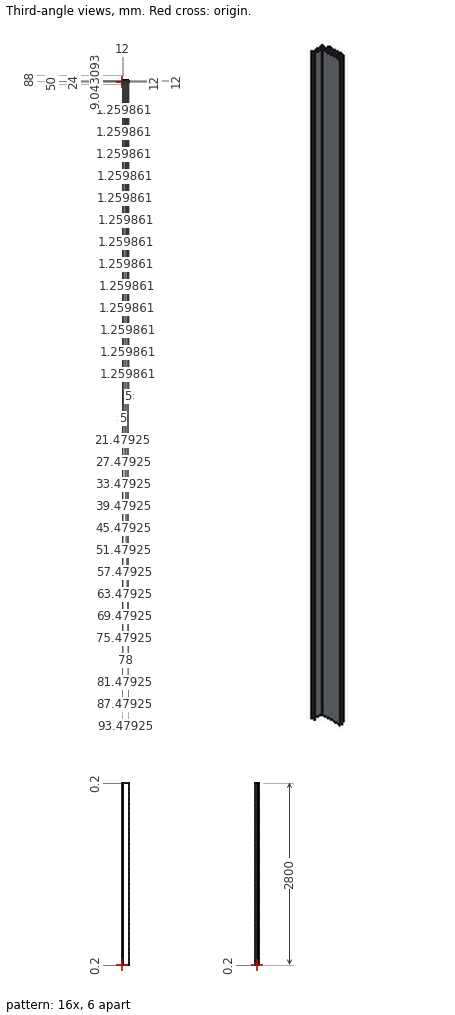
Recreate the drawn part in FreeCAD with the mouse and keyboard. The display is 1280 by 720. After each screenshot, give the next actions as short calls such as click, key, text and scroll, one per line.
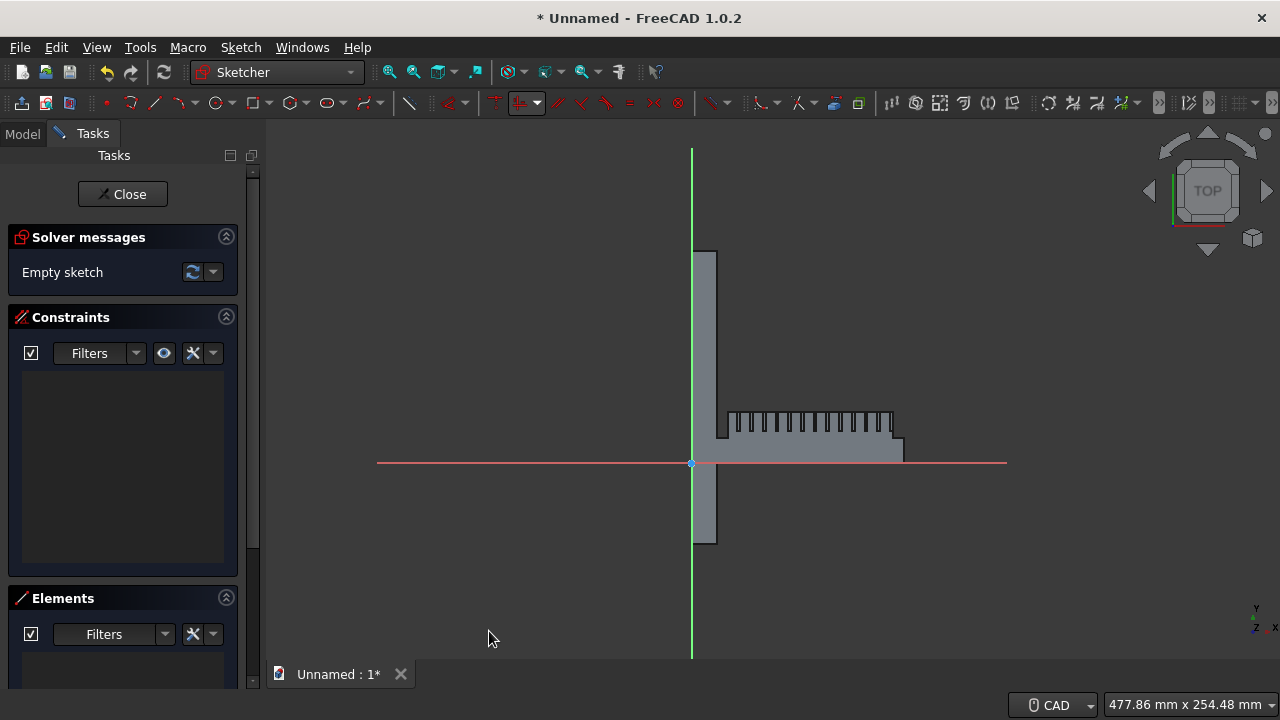
scroll(705, 292, up, 2)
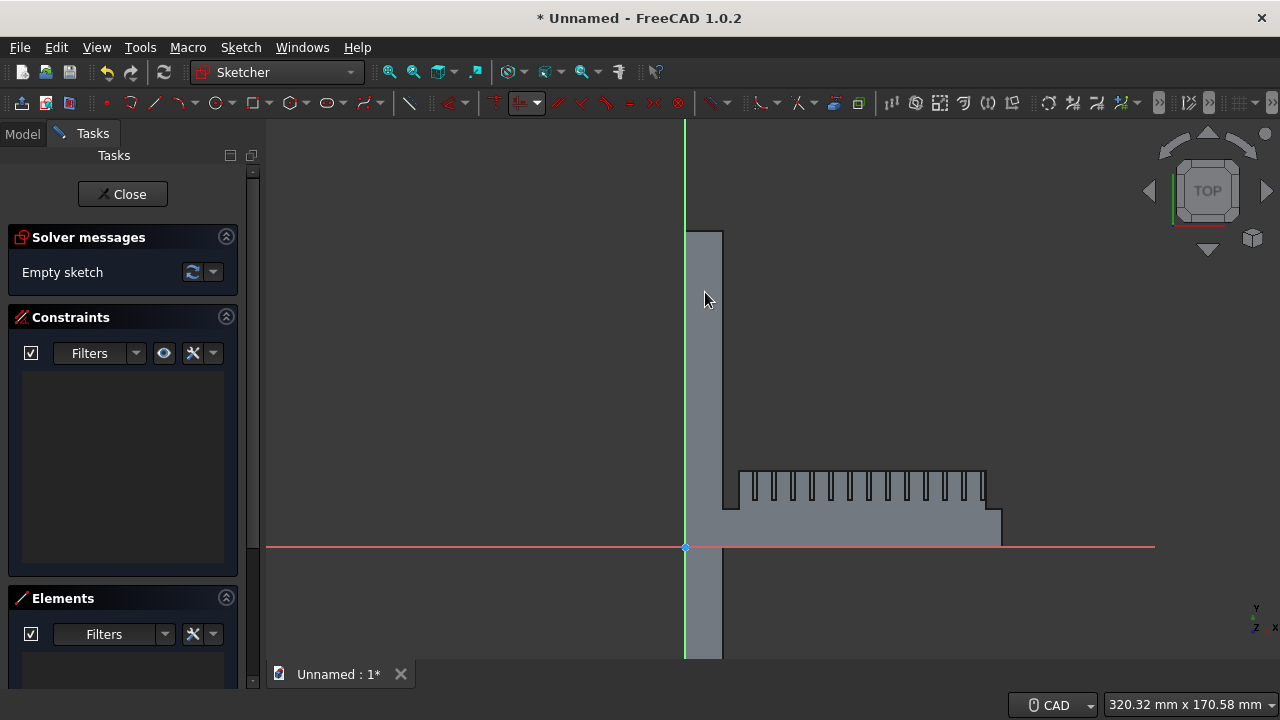
click(254, 104)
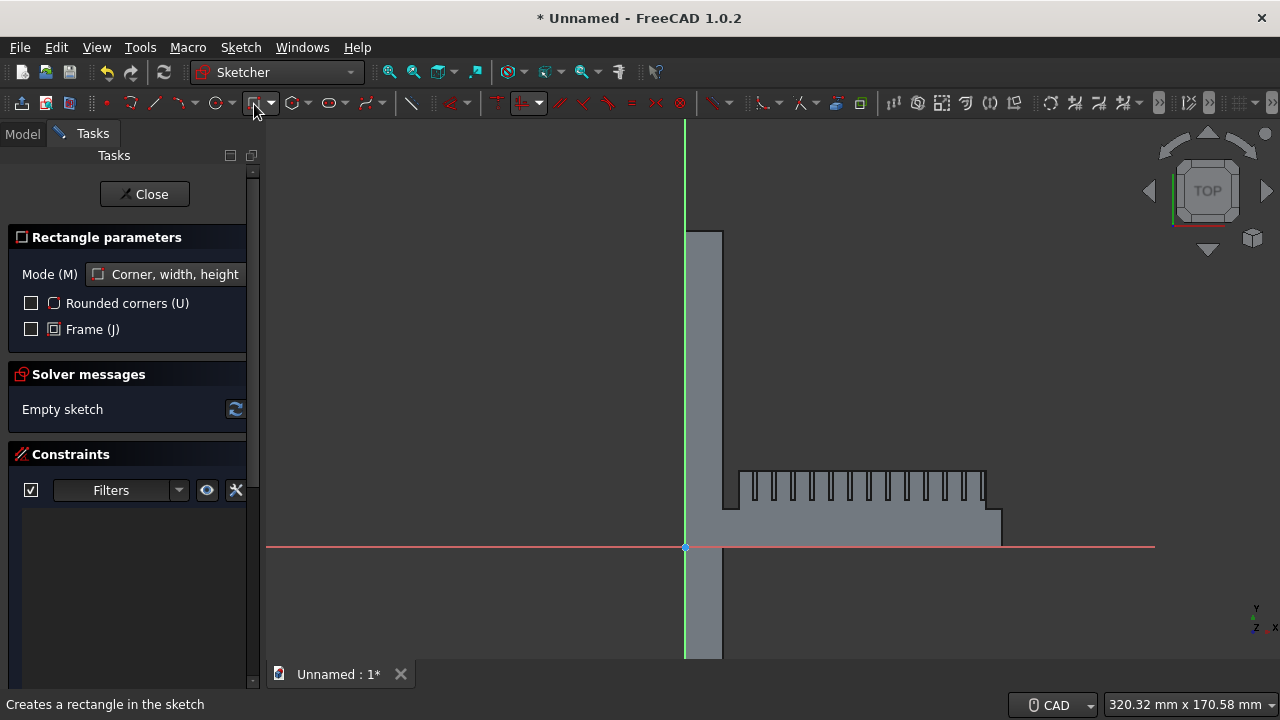
click(685, 231)
move(723, 509)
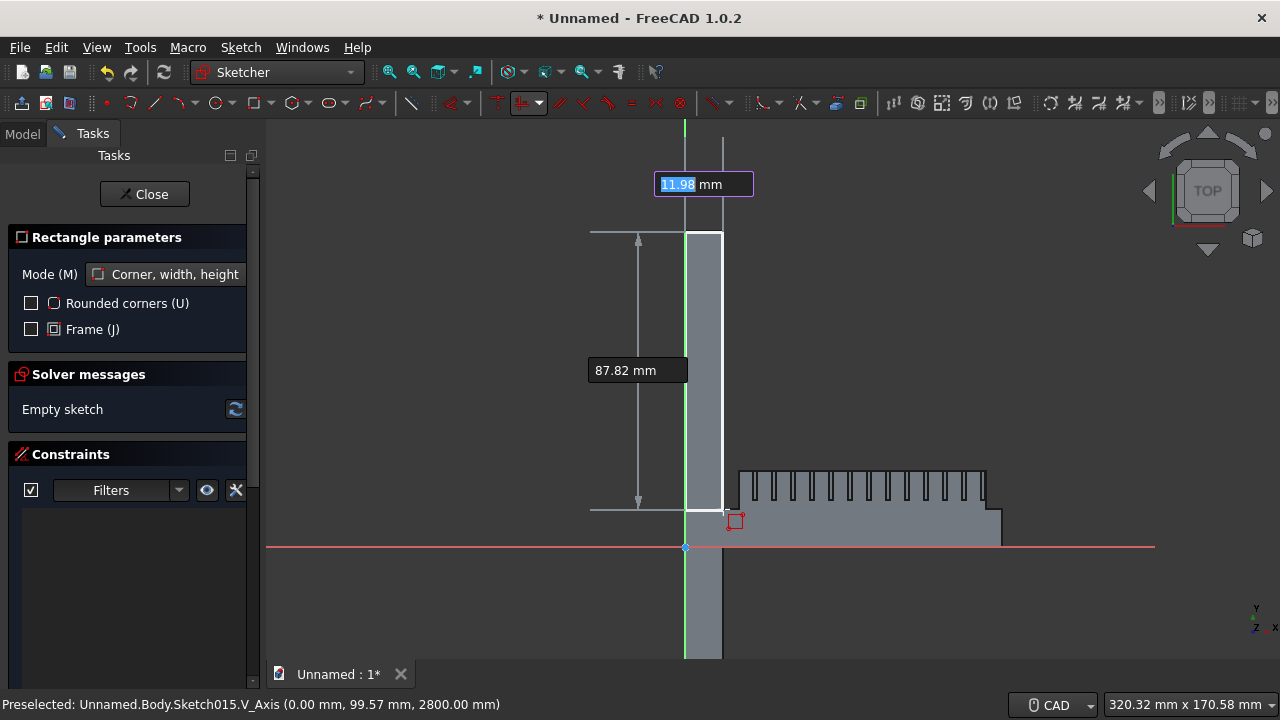
text(12)
key(Tab)
text(88)
key(Return)
key(Escape)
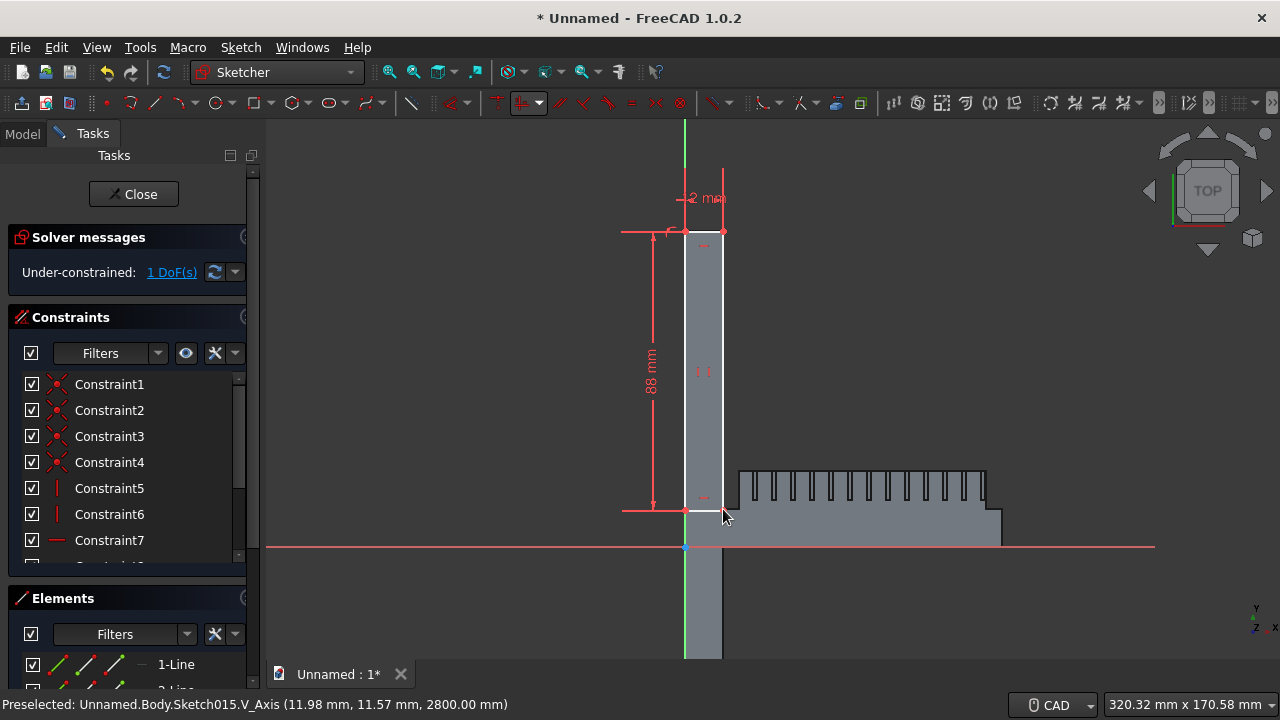
click(450, 104)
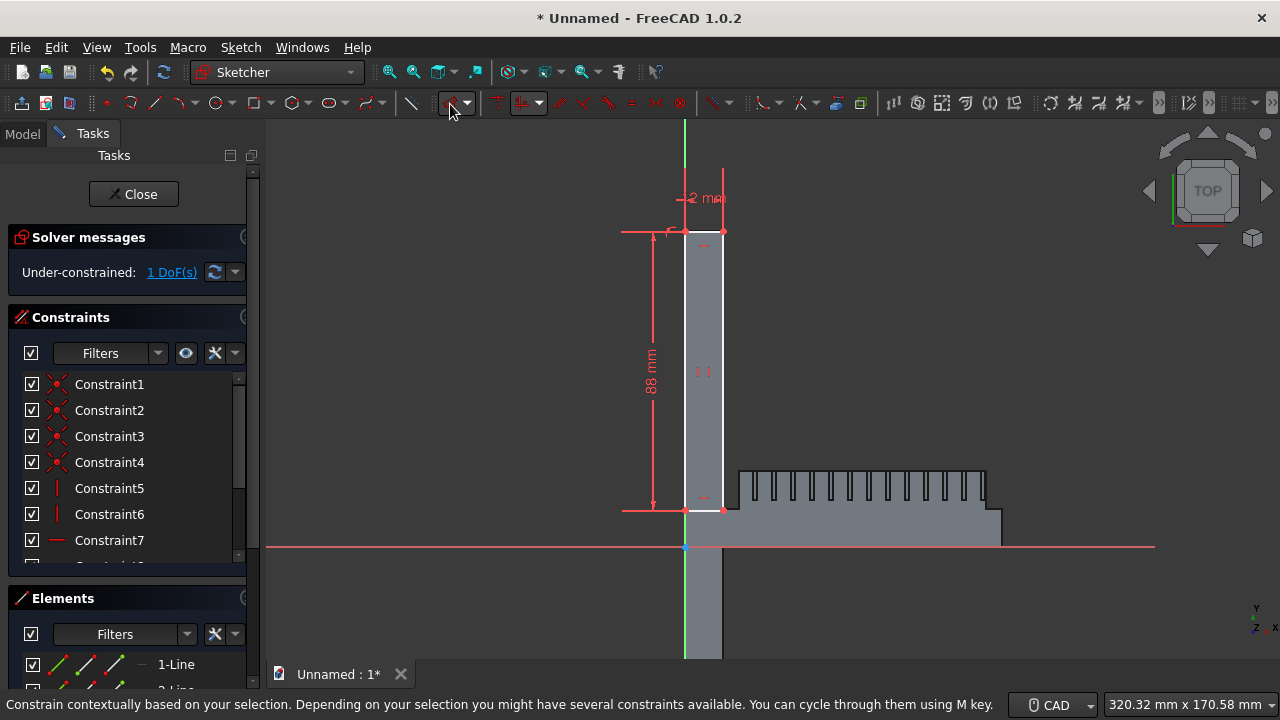
click(685, 511)
click(651, 529)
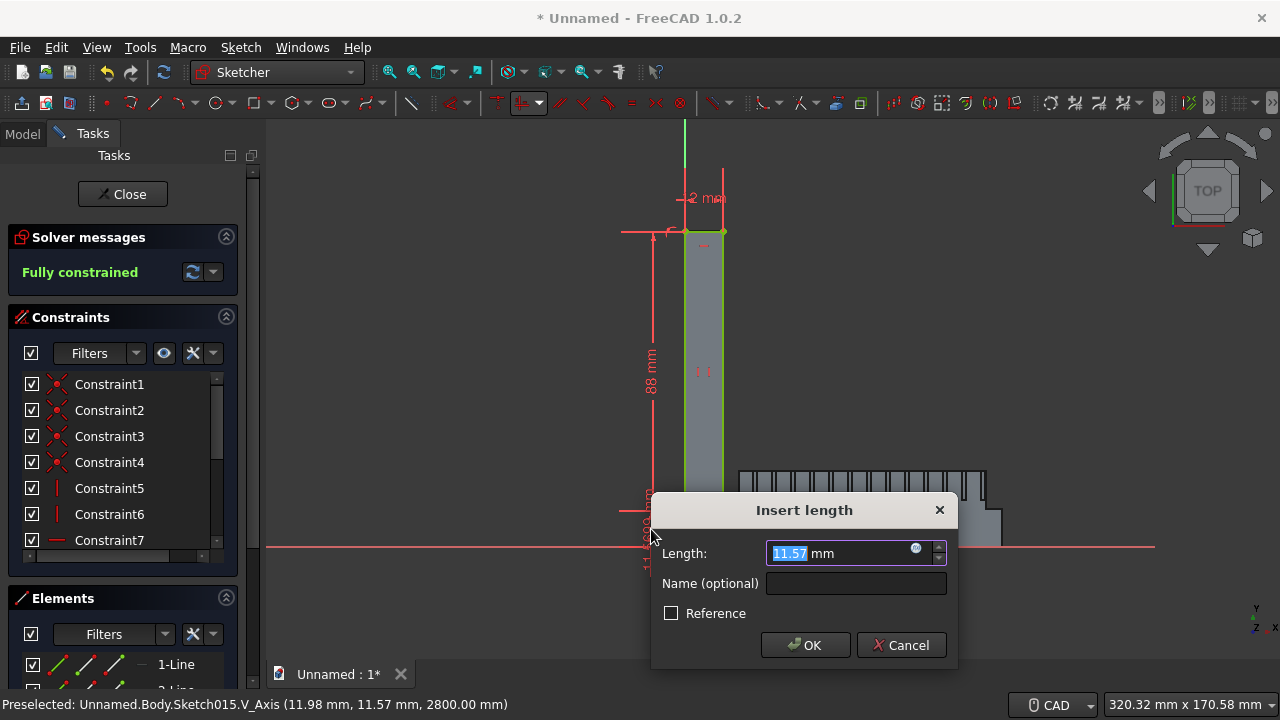
text(12)
key(Return)
key(Escape)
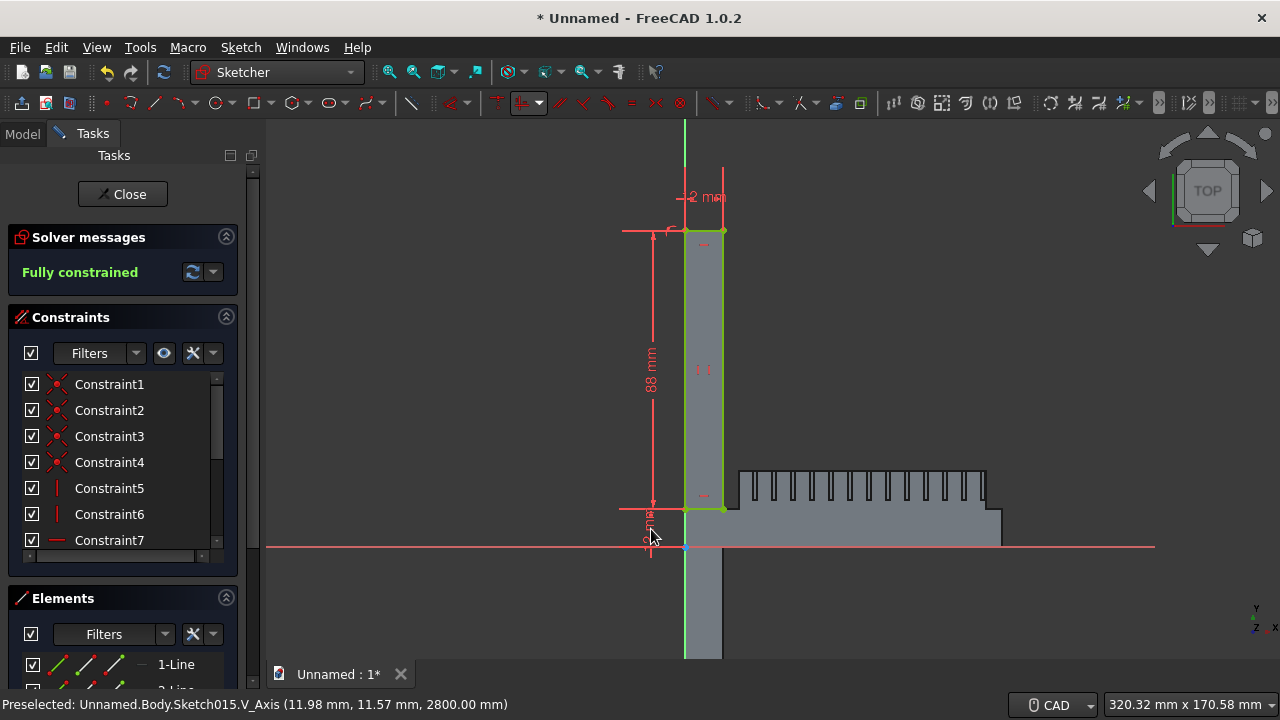
click(123, 194)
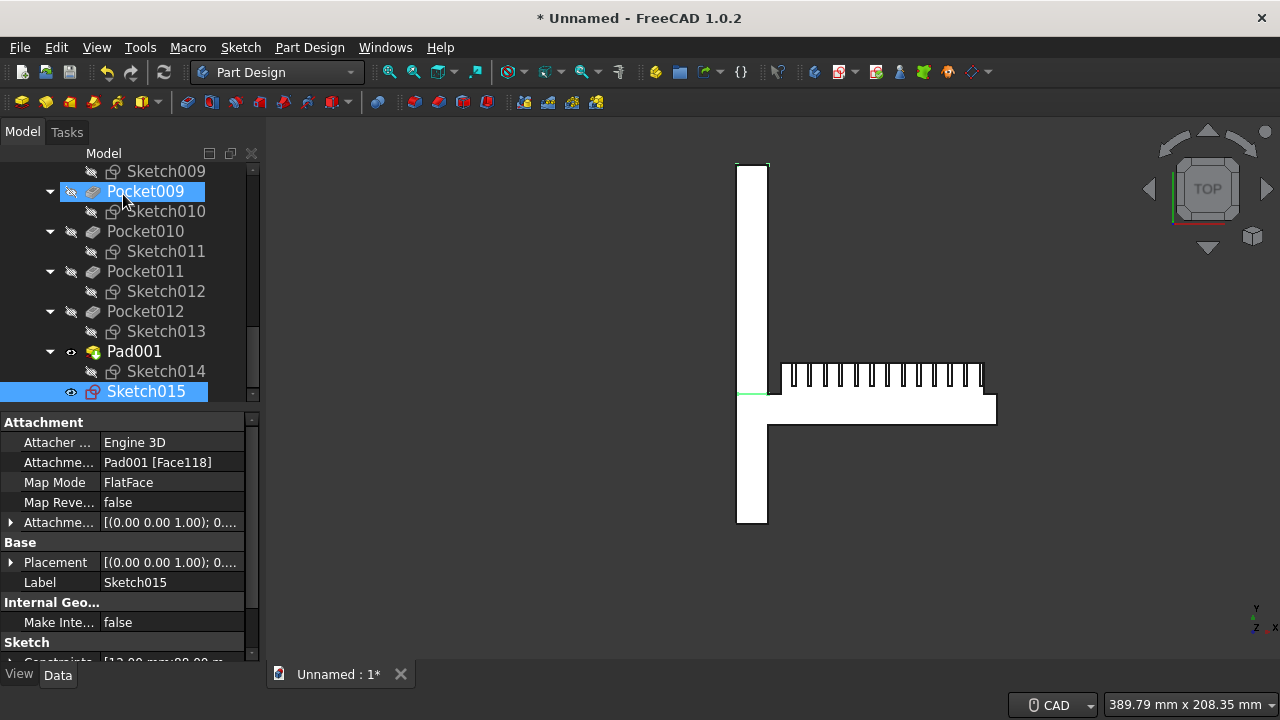
click(188, 102)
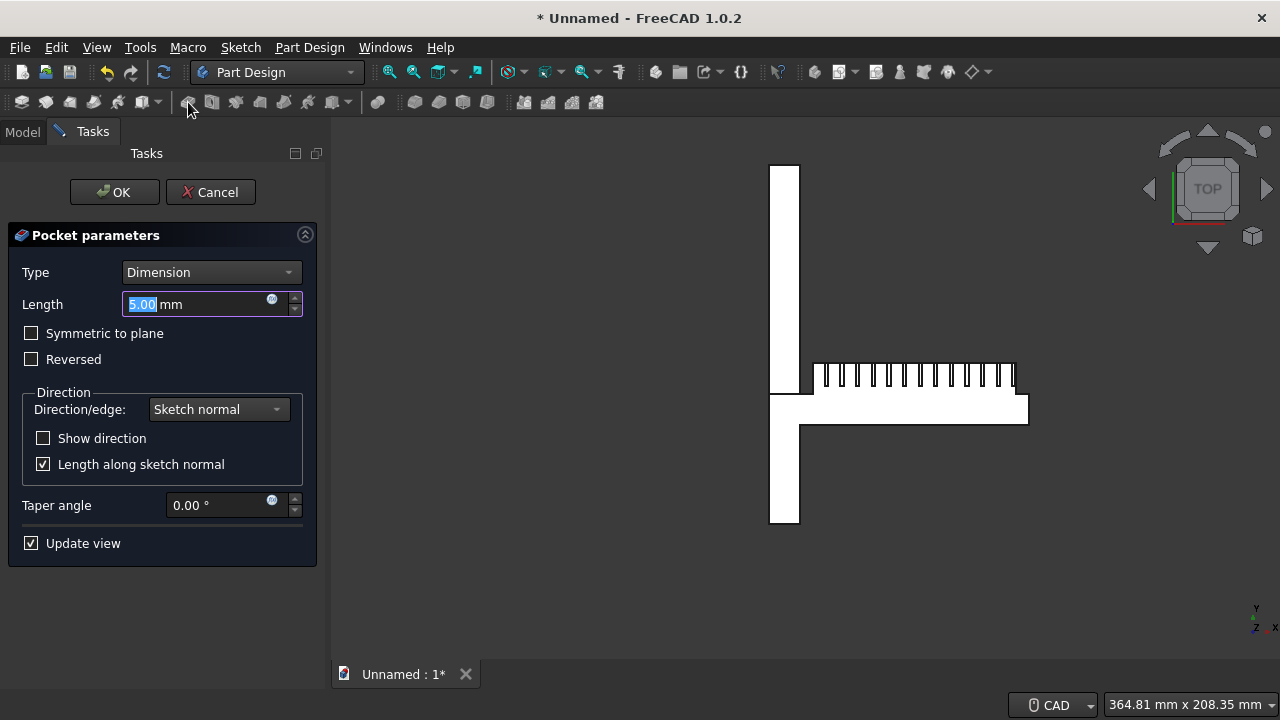
click(212, 272)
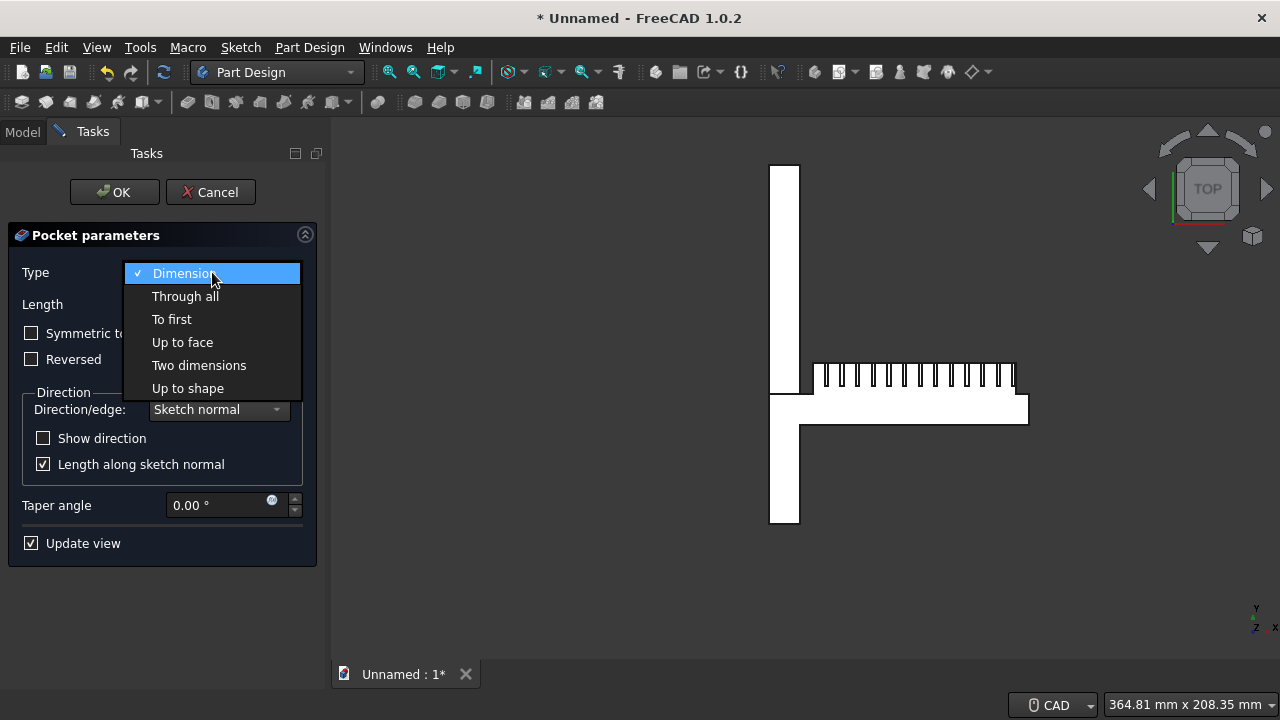
click(212, 296)